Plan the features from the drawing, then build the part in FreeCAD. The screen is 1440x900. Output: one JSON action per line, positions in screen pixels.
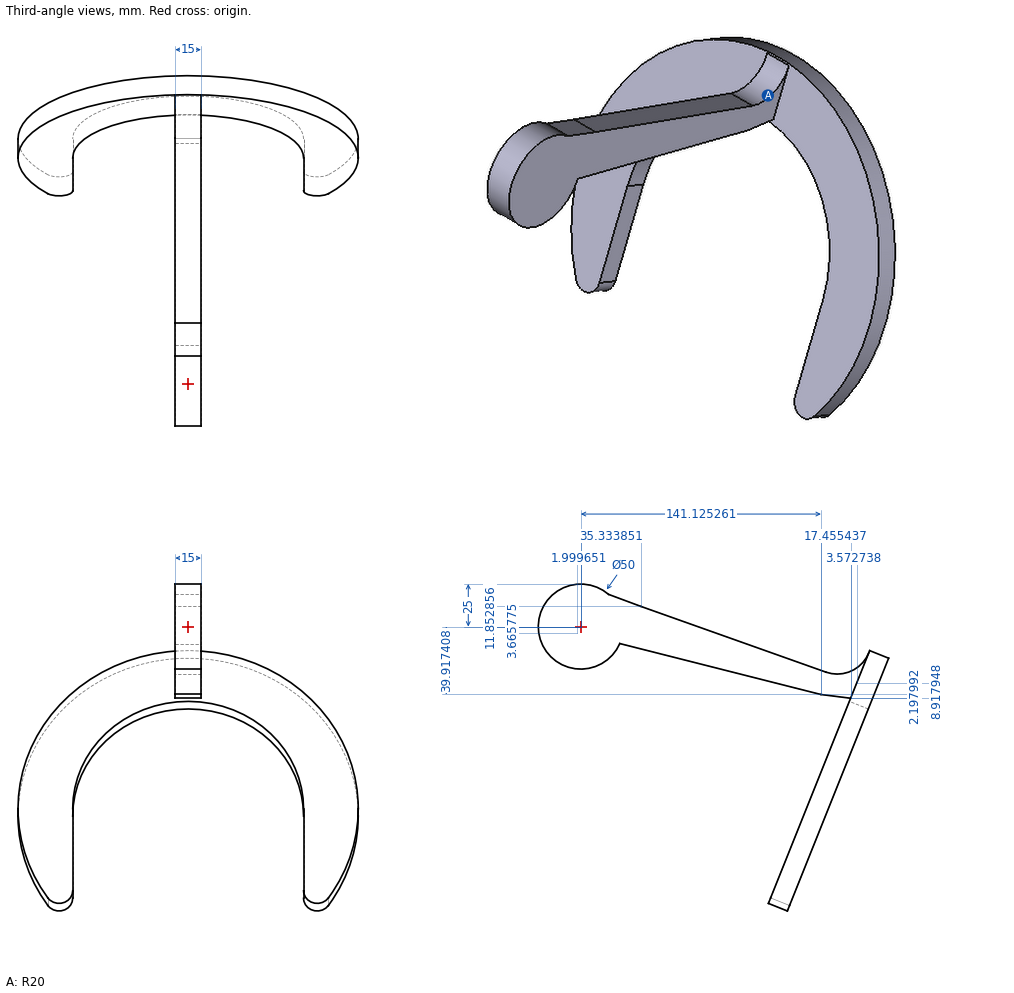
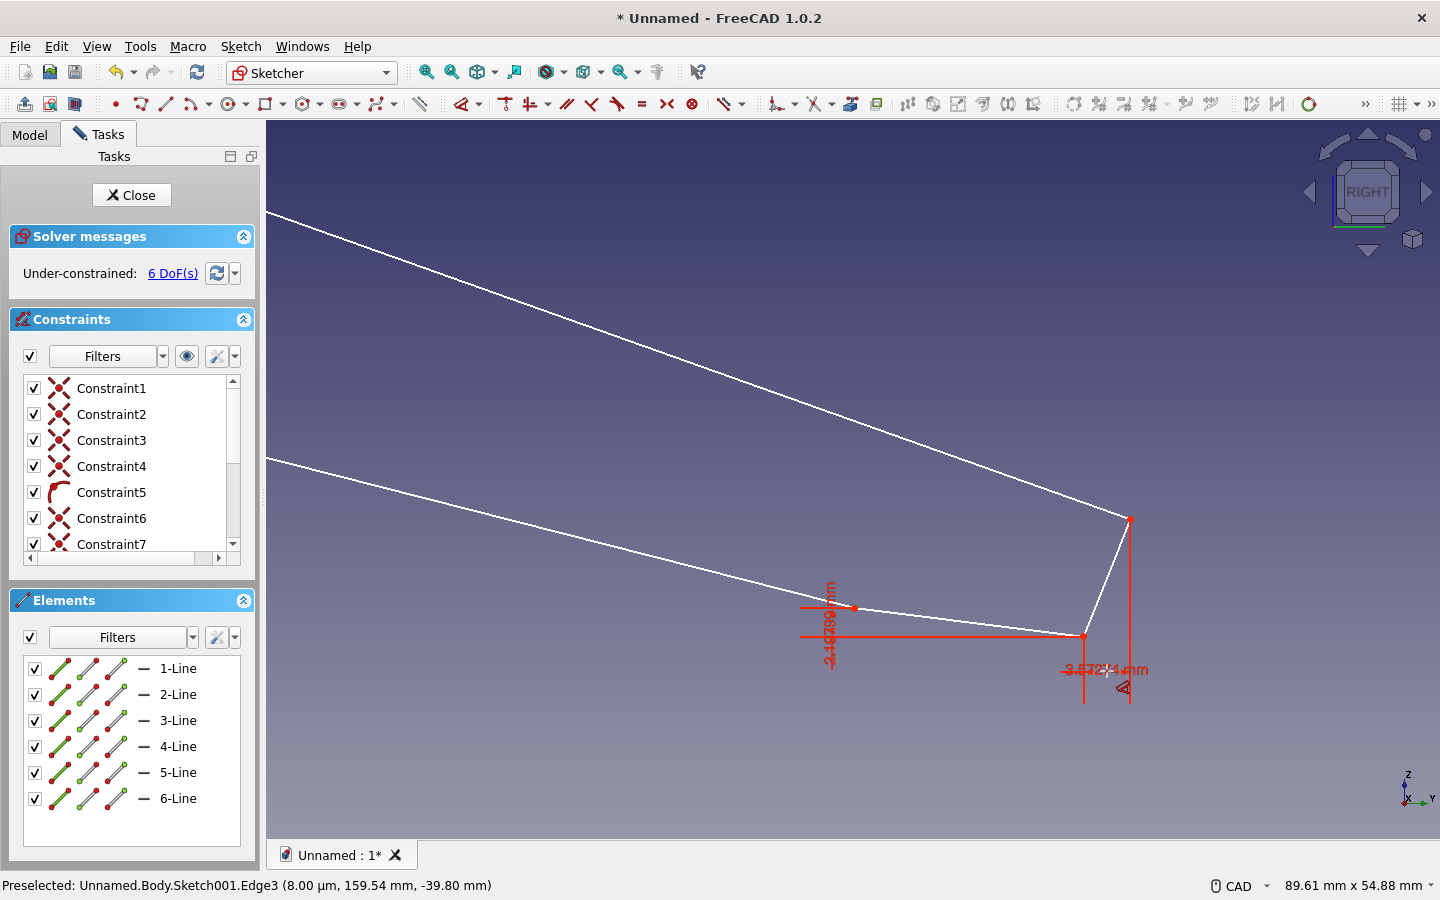
{"action": "left_click", "coordinate": [1098, 602]}
{"action": "left_click", "coordinate": [1164, 578]}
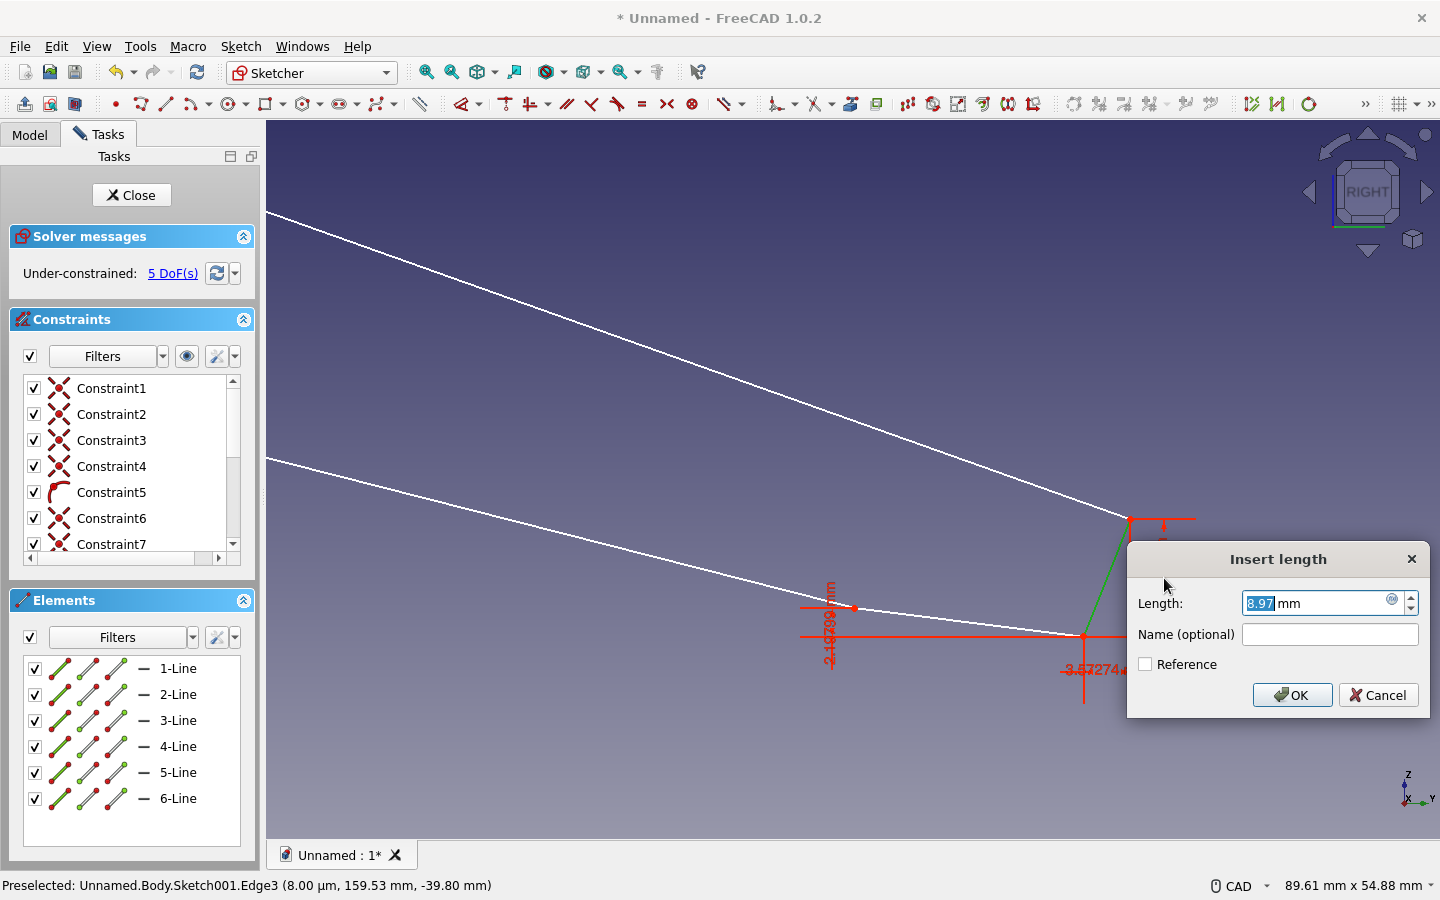
{"action": "type", "text": "8.917948"}
{"action": "key", "text": "Return"}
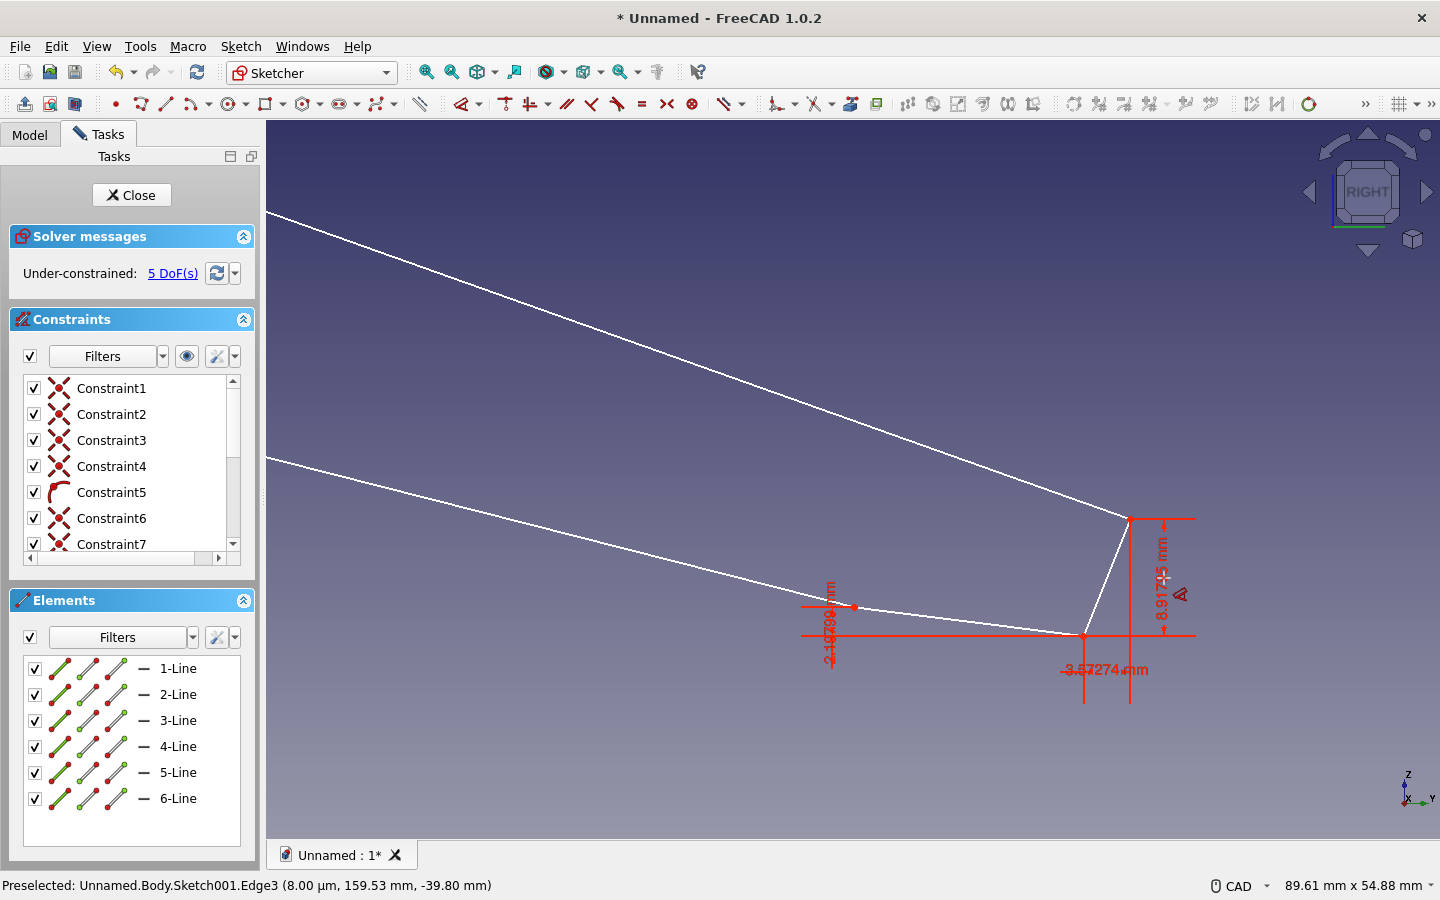
{"action": "left_click", "coordinate": [855, 607]}
{"action": "left_click", "coordinate": [889, 378]}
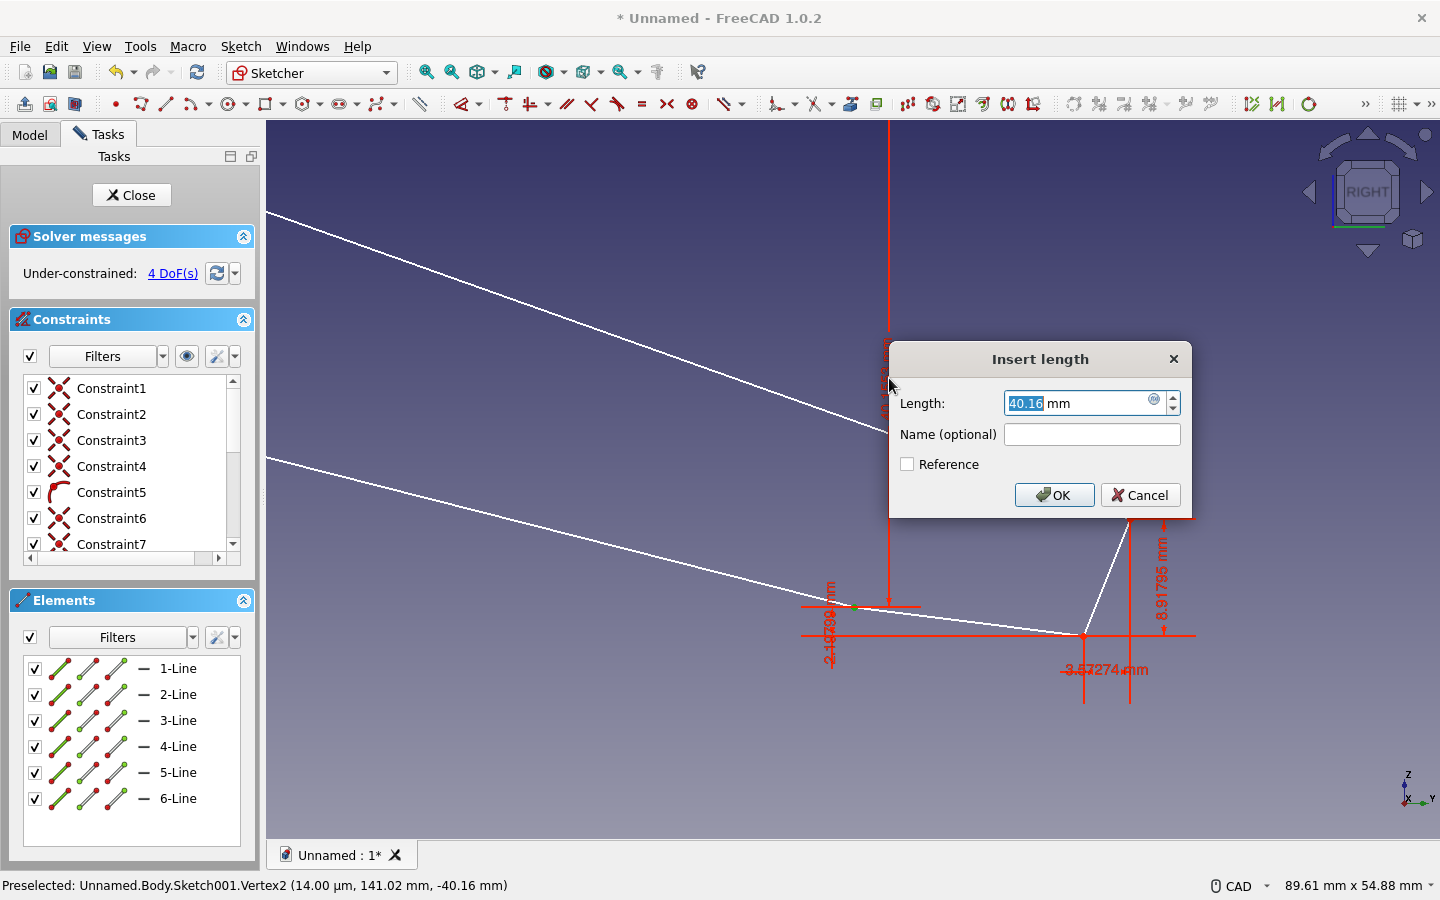
{"action": "type", "text": "39.917408"}
{"action": "key", "text": "Return"}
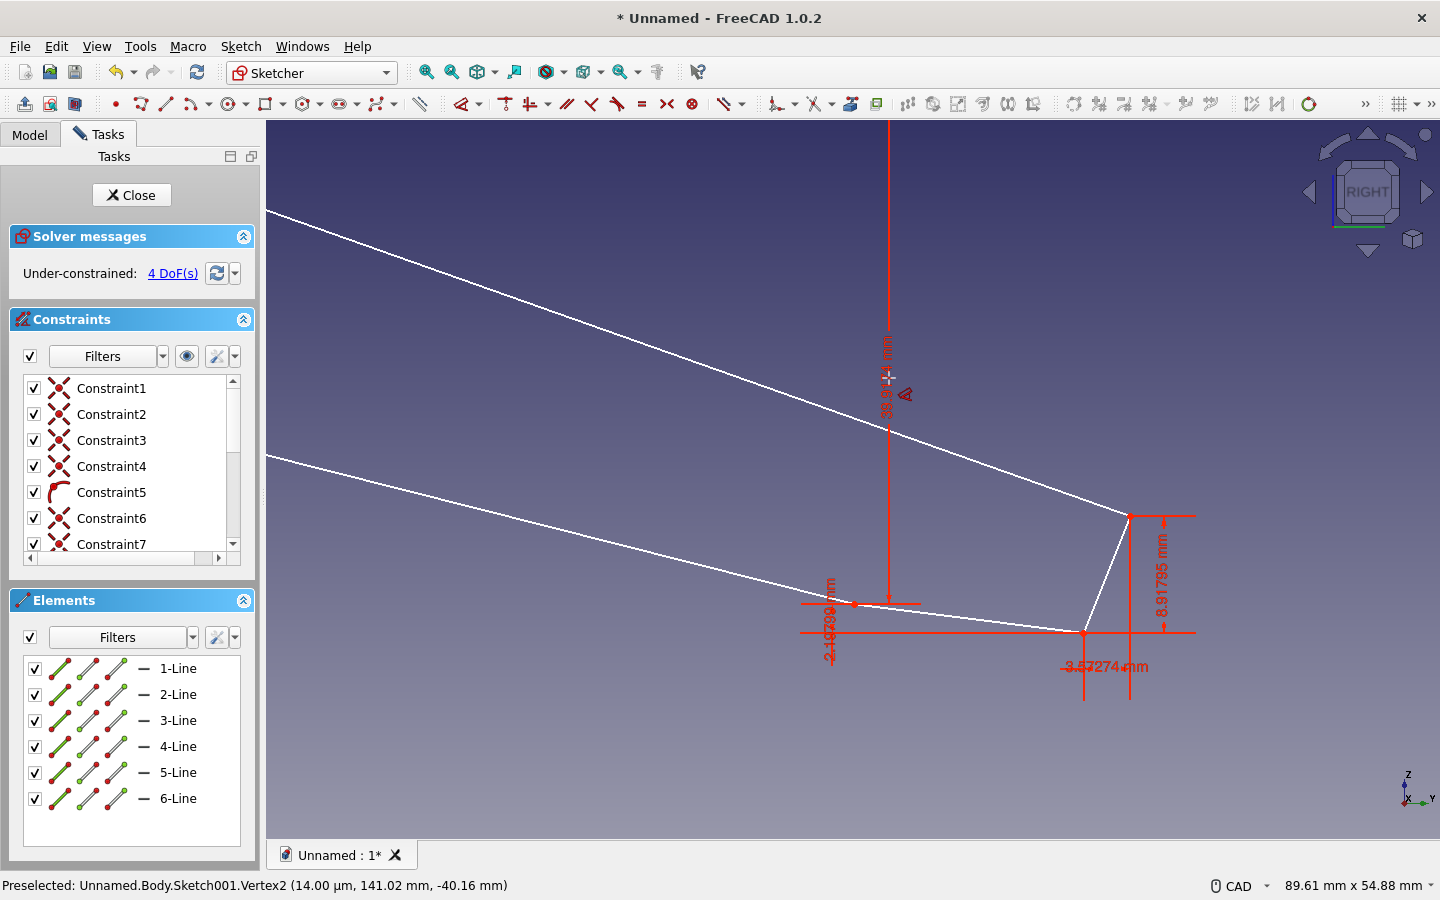
{"action": "scroll", "coordinate": [1098, 603], "scroll_direction": "down", "scroll_amount": 6}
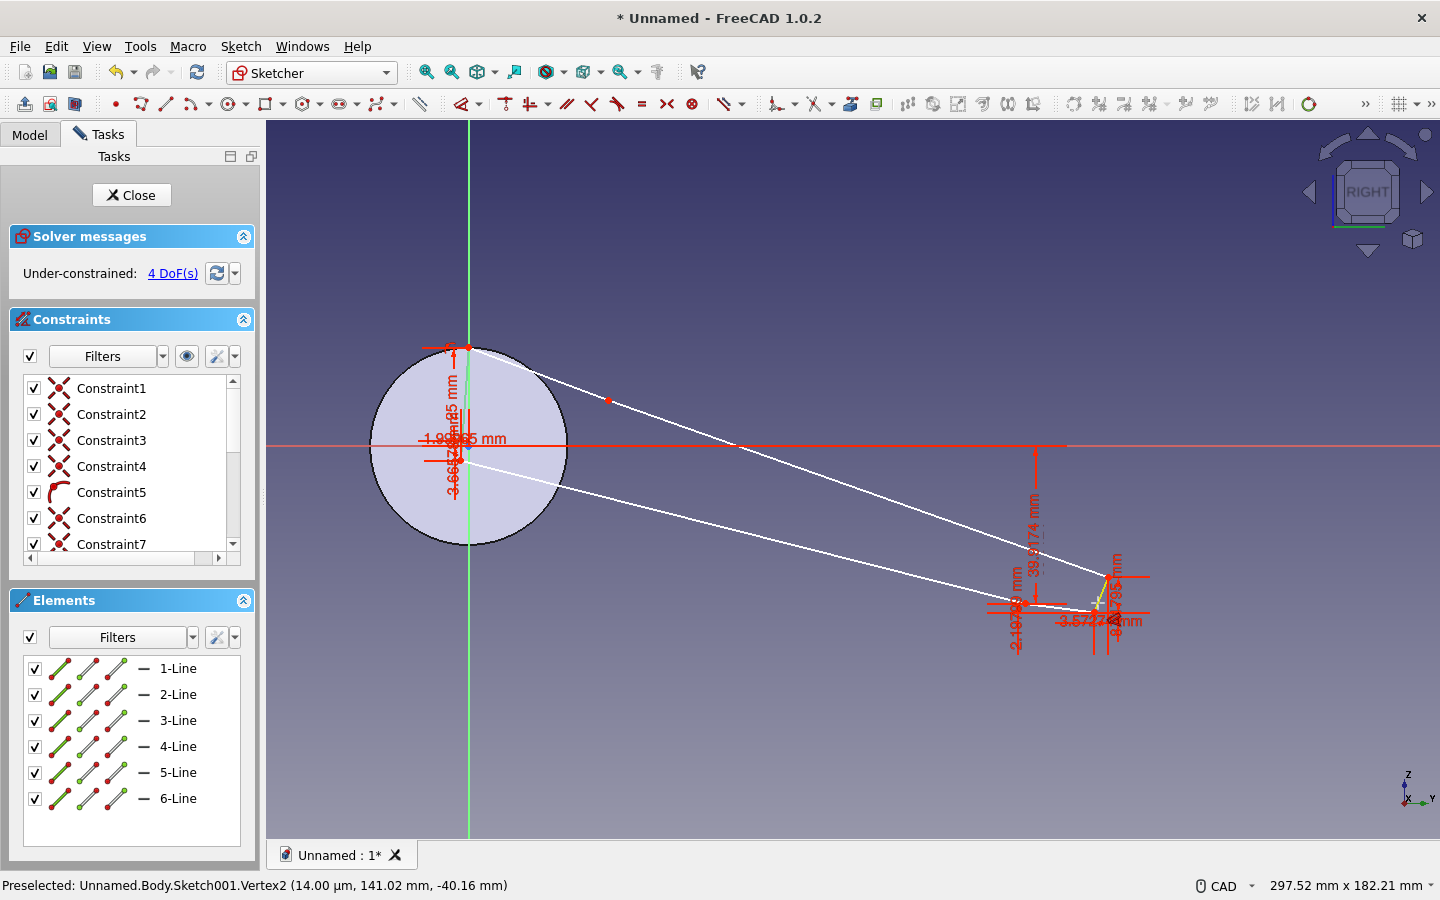
{"action": "left_click", "coordinate": [608, 400]}
{"action": "left_click", "coordinate": [571, 366]}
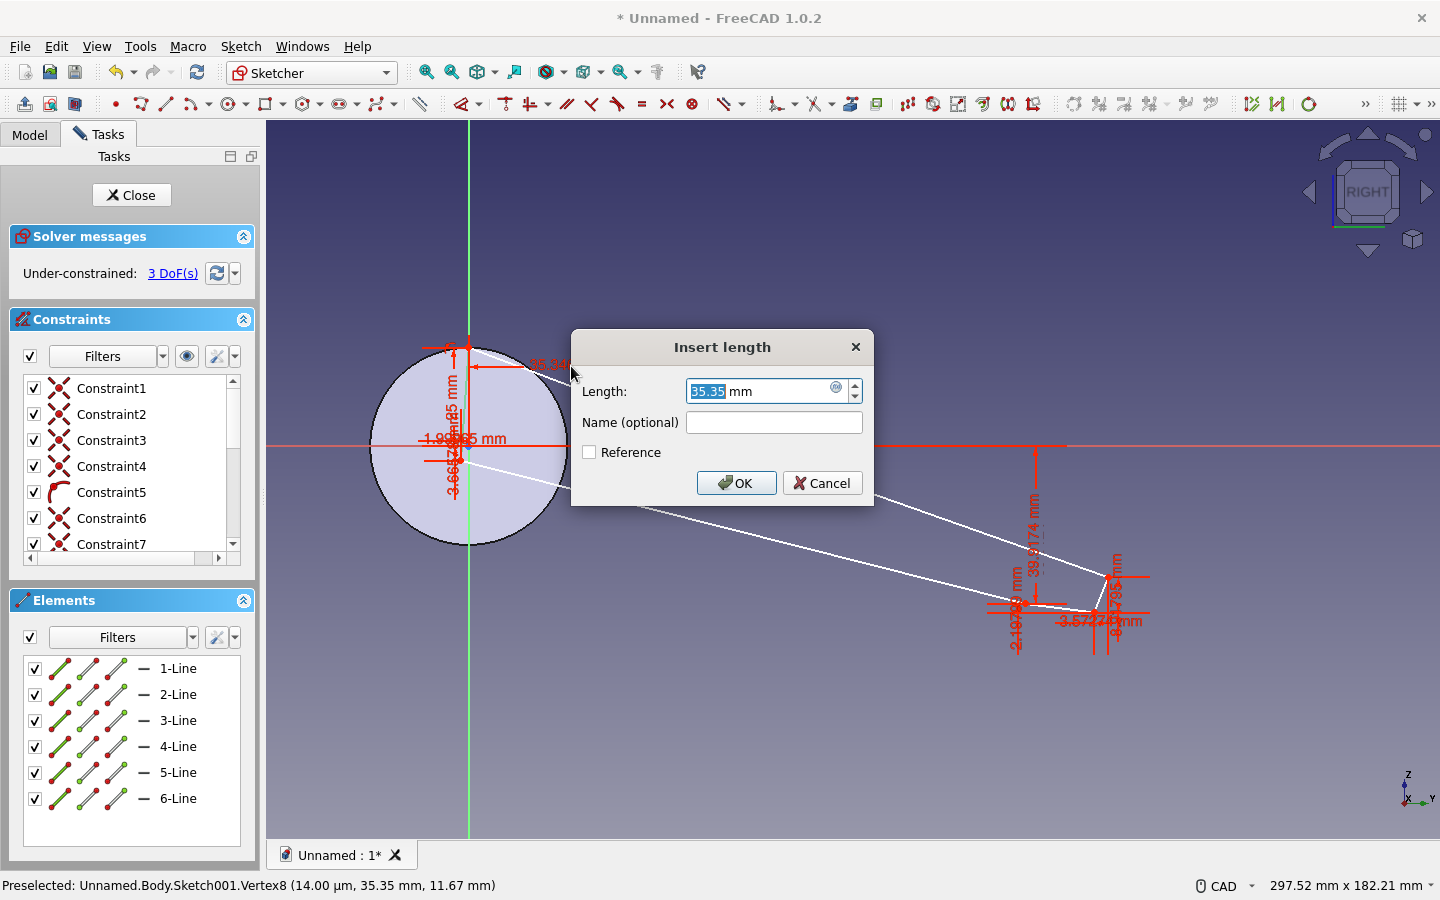
{"action": "type", "text": "35.333851"}
{"action": "key", "text": "Return"}